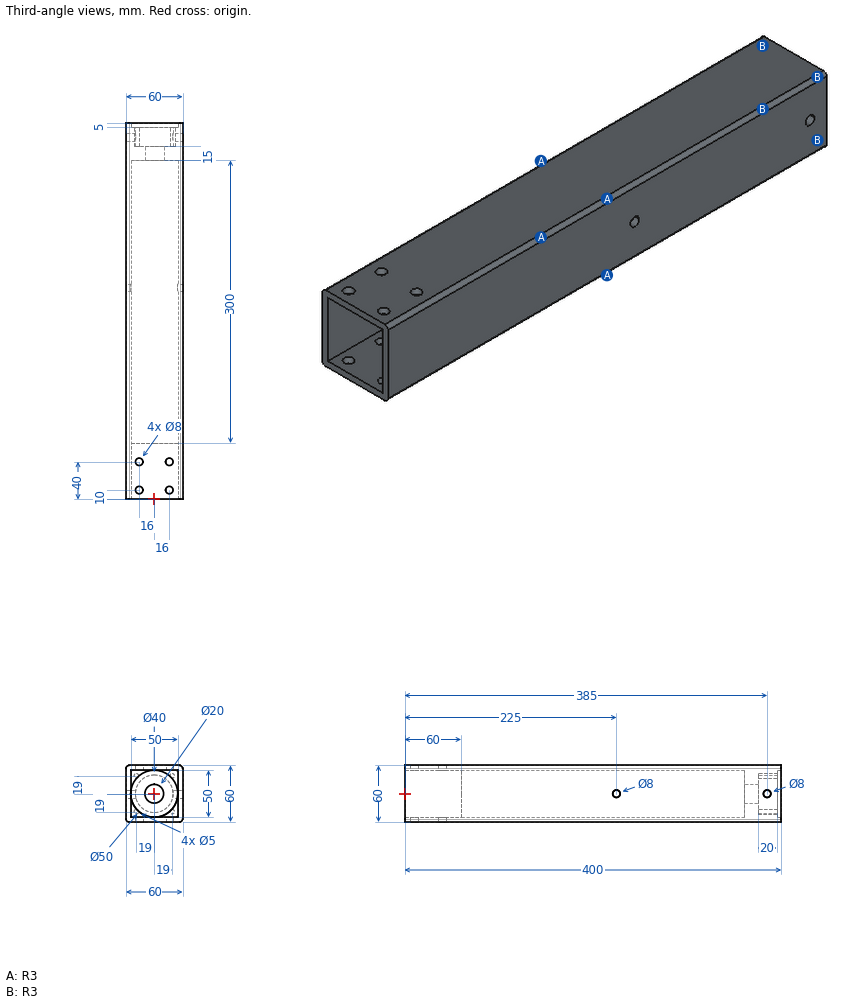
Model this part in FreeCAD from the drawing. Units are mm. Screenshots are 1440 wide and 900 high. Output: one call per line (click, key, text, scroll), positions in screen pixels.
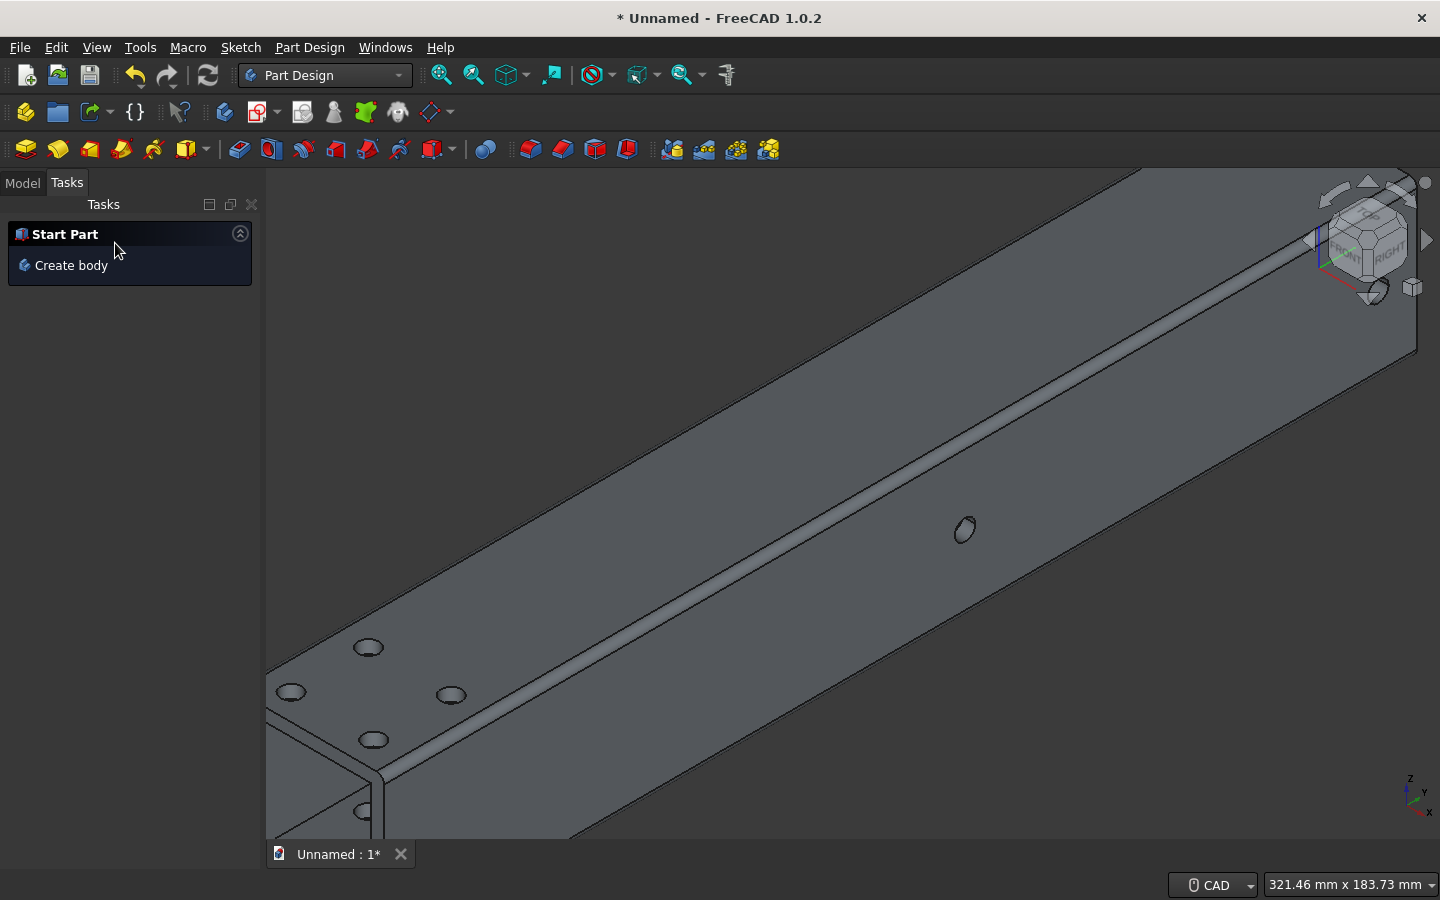
click(442, 76)